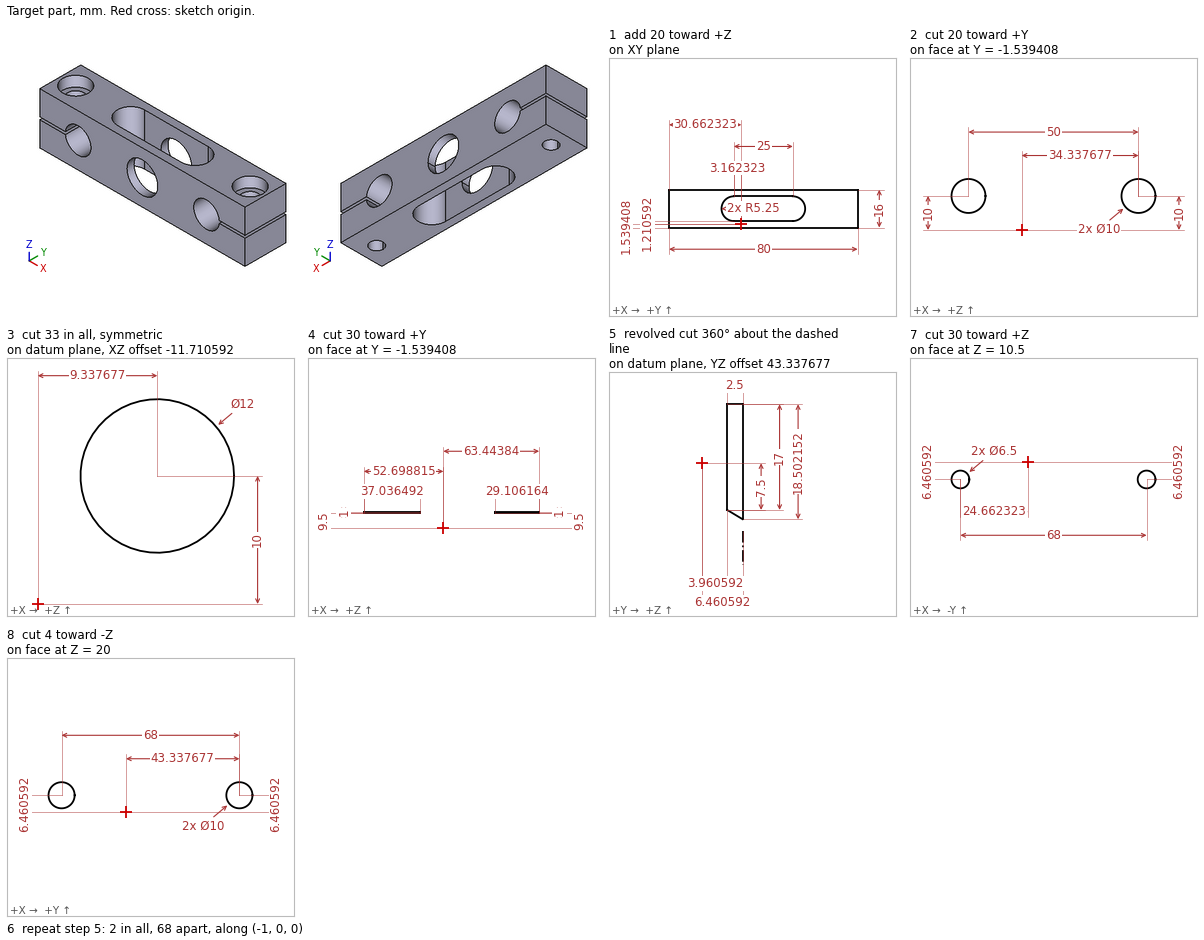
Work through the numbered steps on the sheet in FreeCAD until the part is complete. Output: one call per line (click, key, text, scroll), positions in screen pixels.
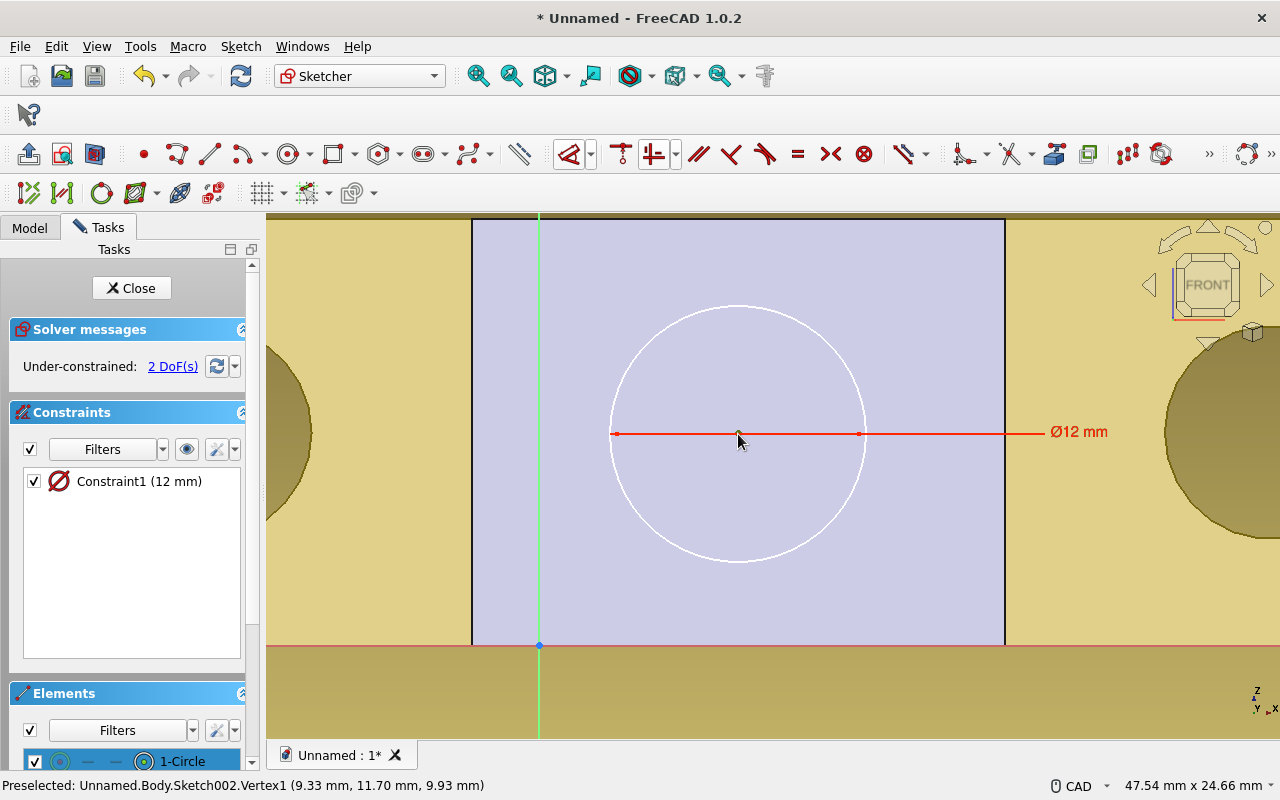
key(i)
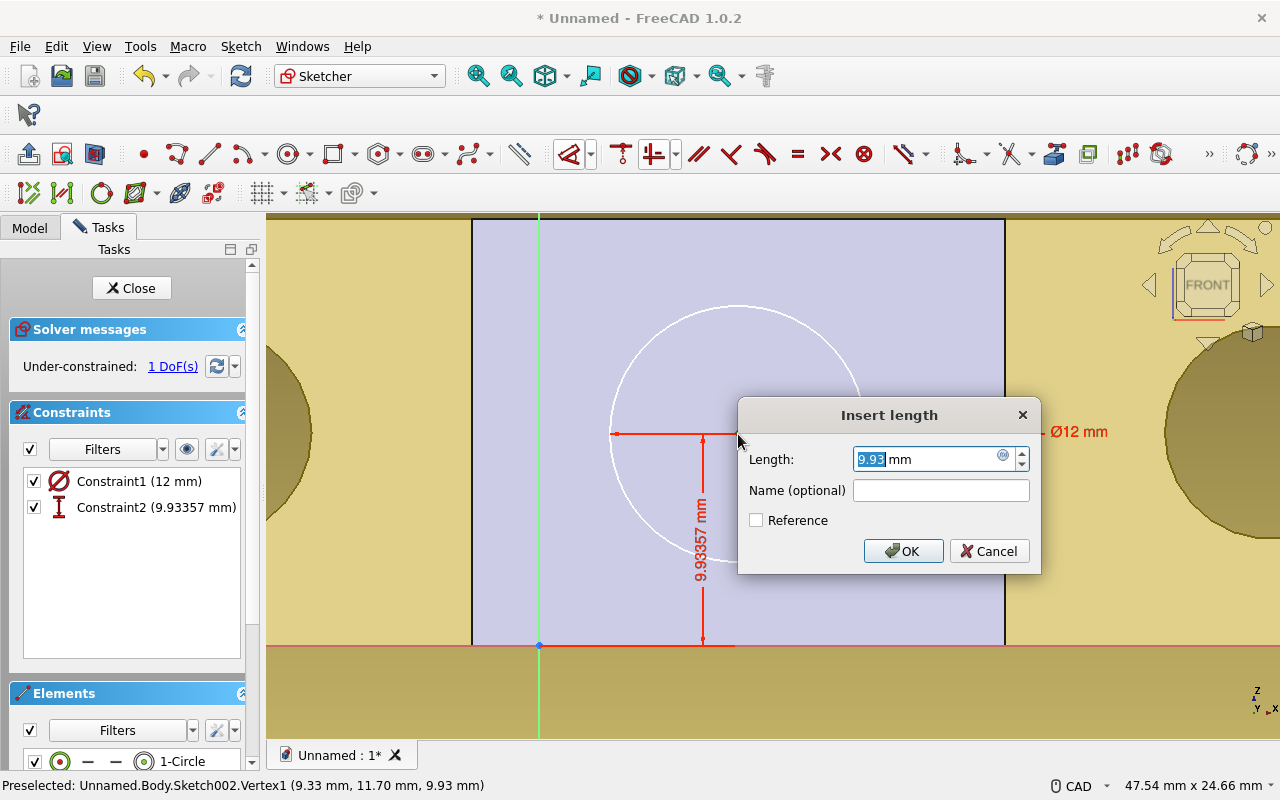
text(10)
key(Return)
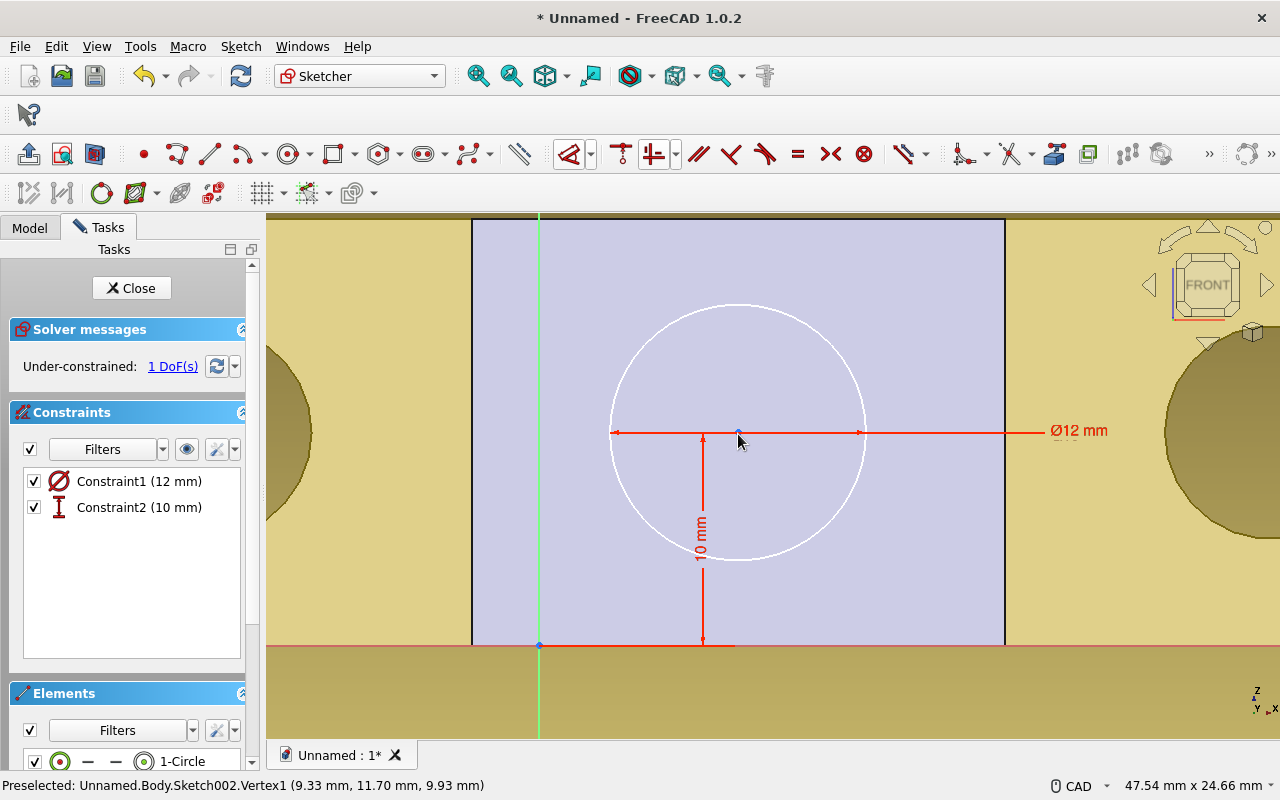
click(738, 433)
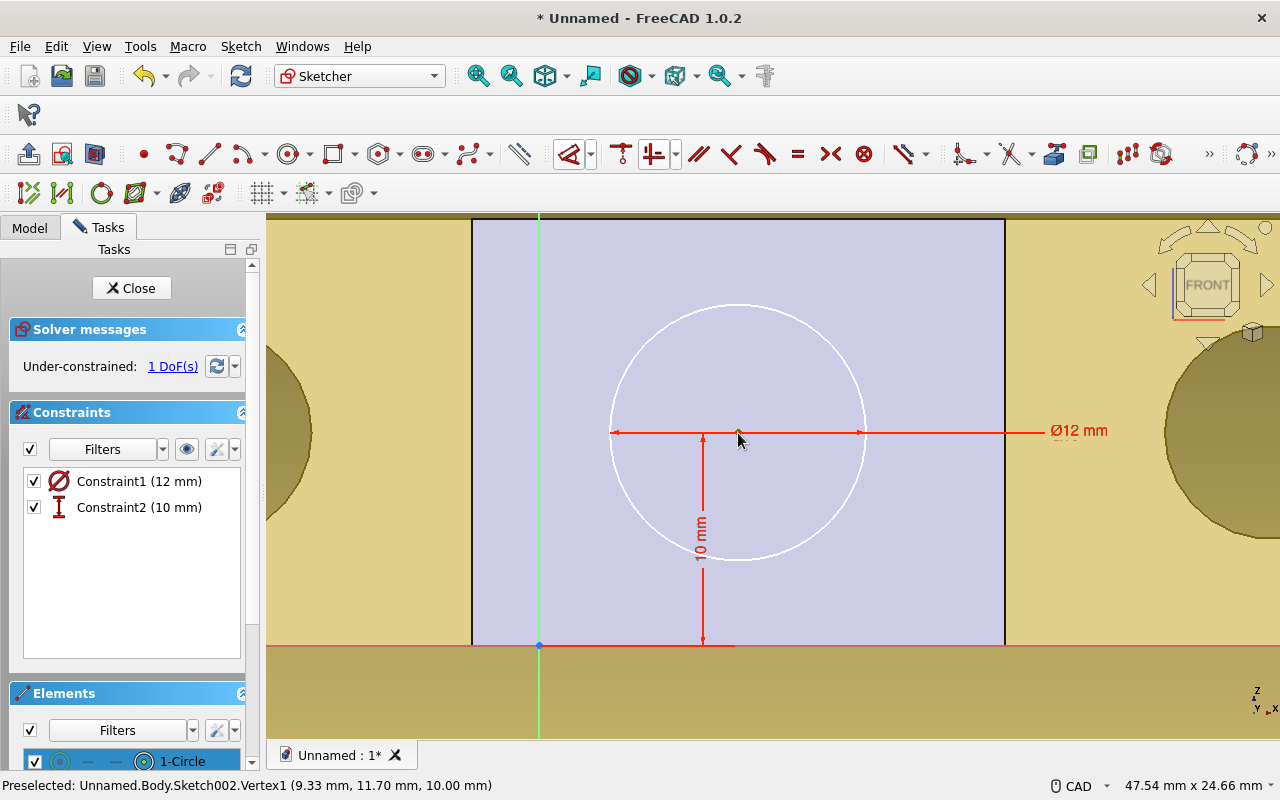
click(590, 154)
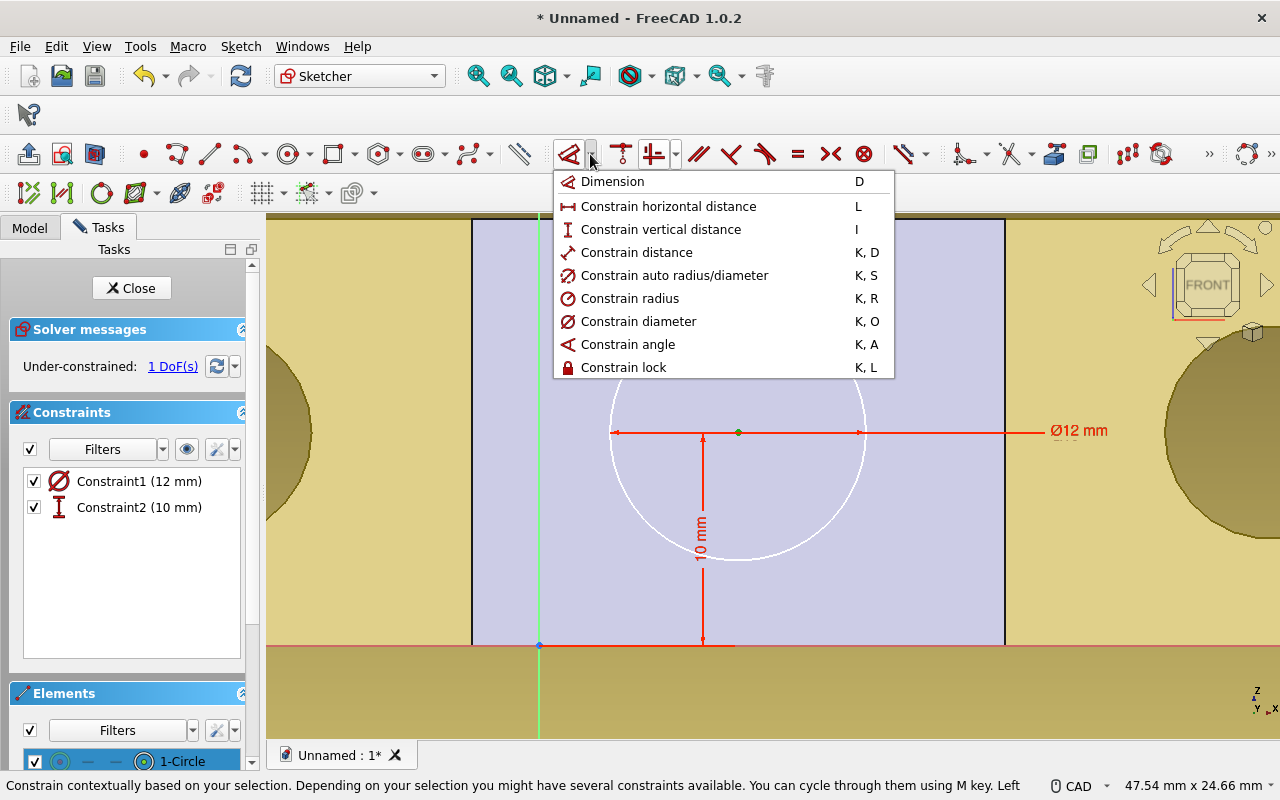
click(724, 206)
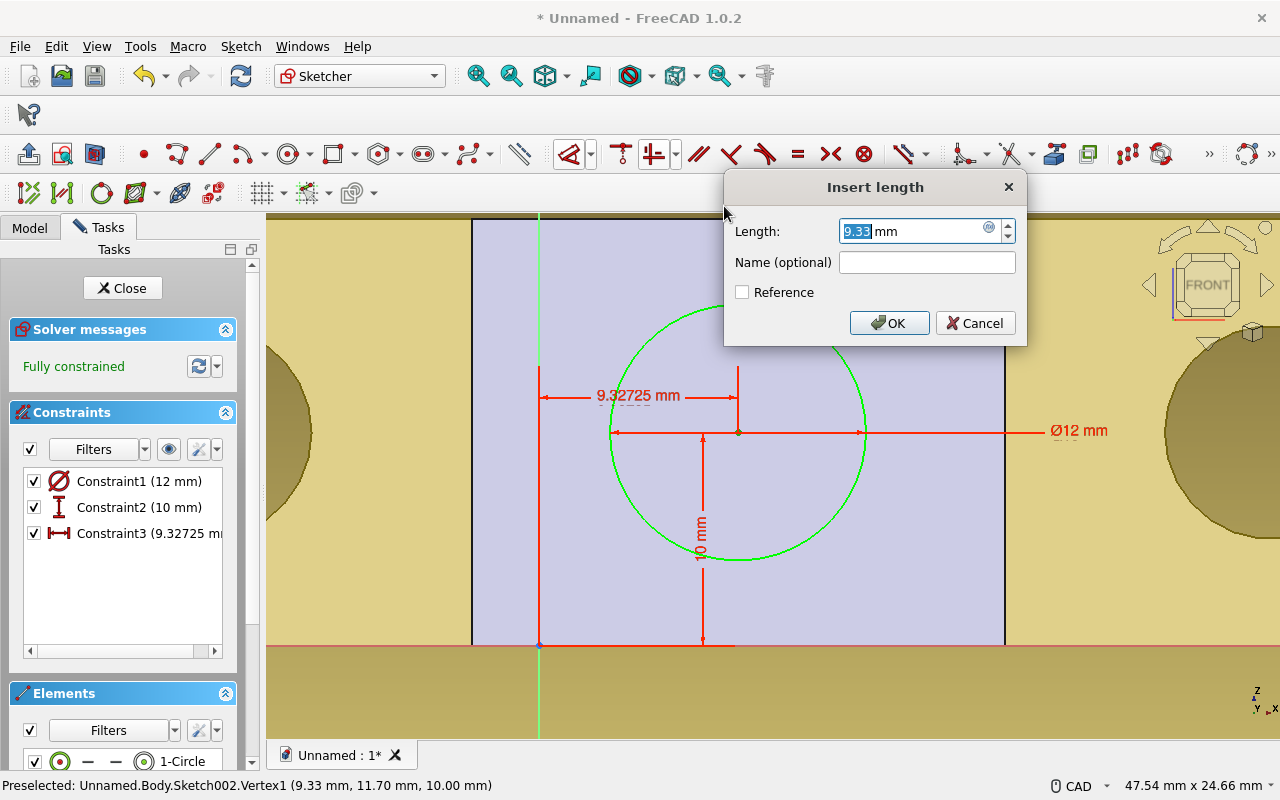
text(9.337677)
key(Return)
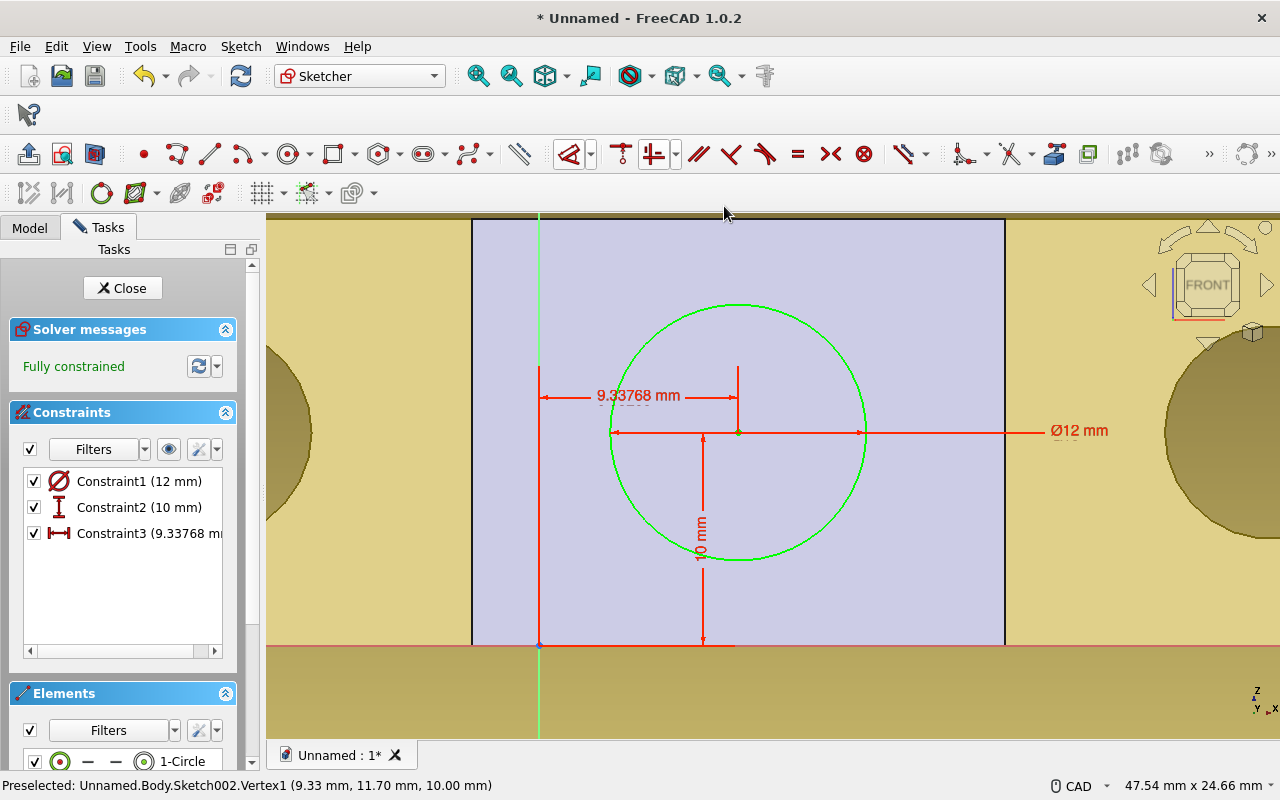
click(123, 288)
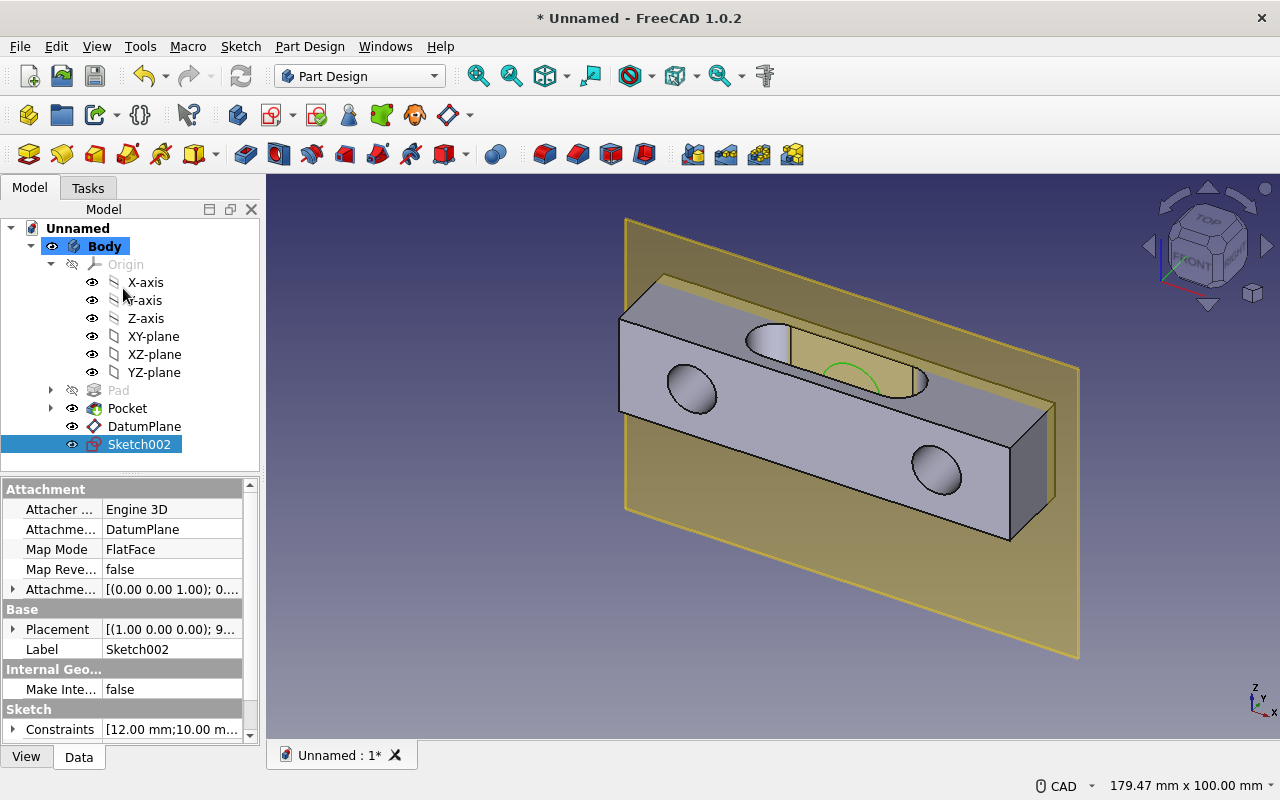
click(246, 154)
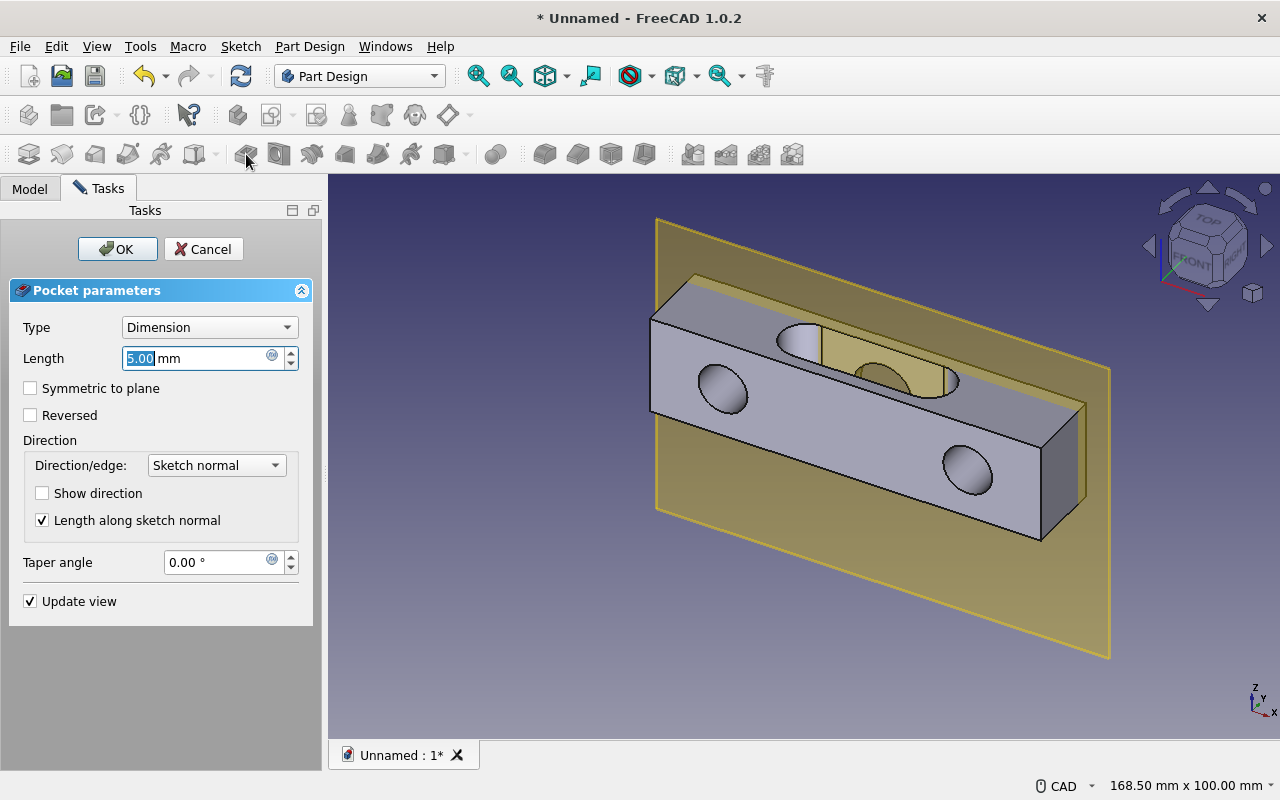
text(33)
key(Tab)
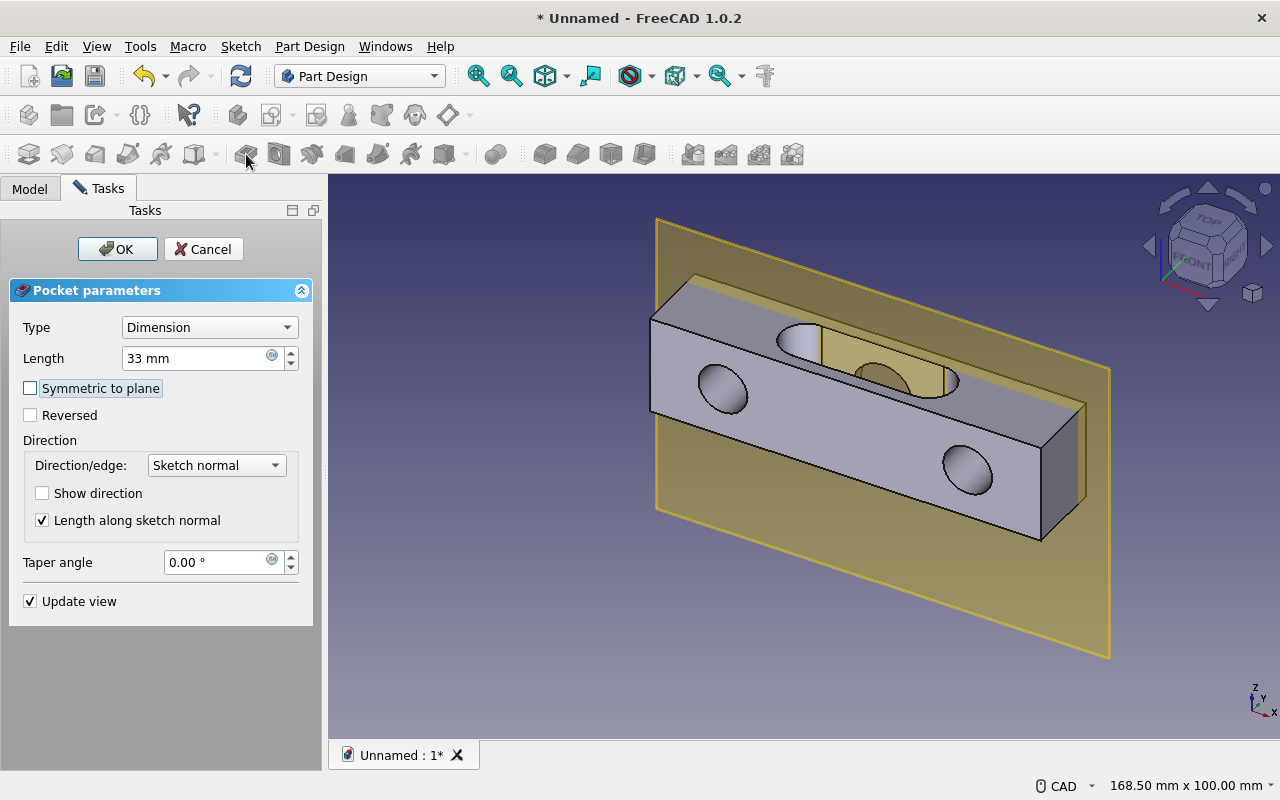
click(31, 388)